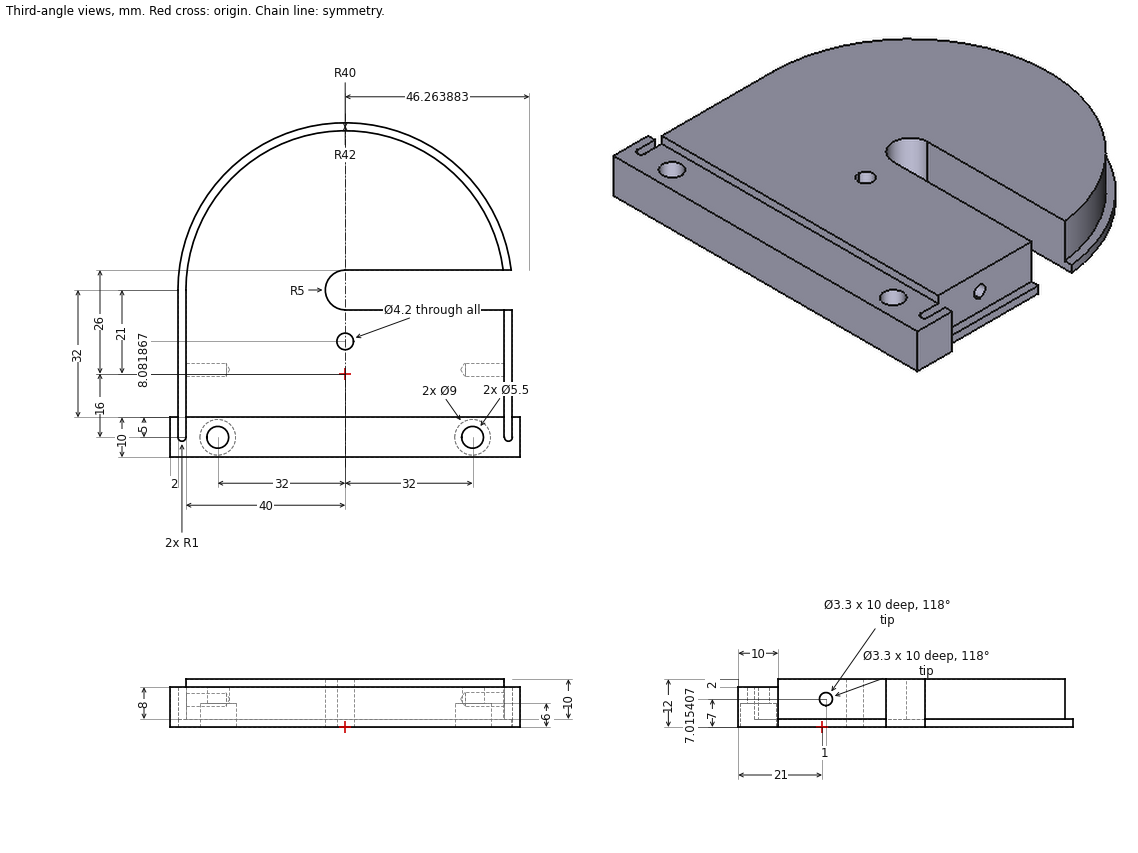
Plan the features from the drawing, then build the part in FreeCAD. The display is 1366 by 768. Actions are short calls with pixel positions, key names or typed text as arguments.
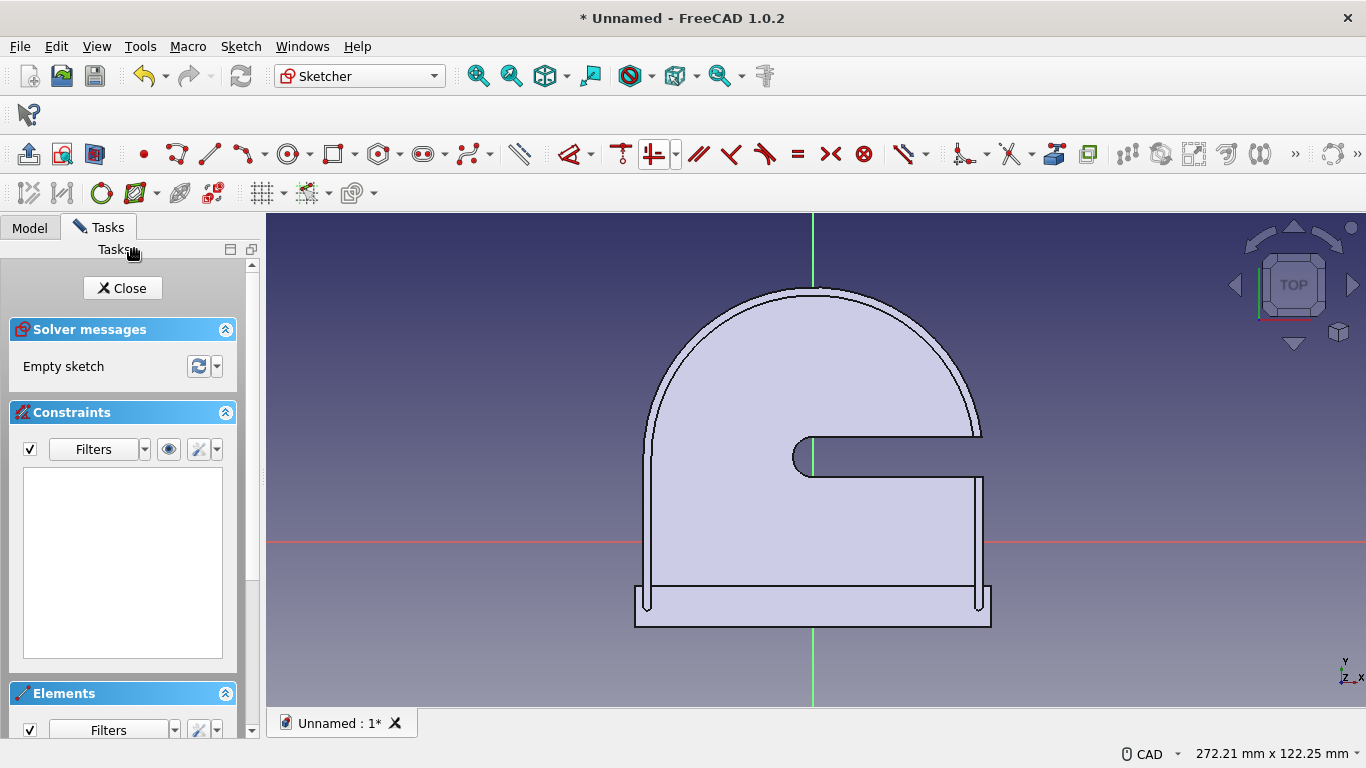
key(q)
key(s)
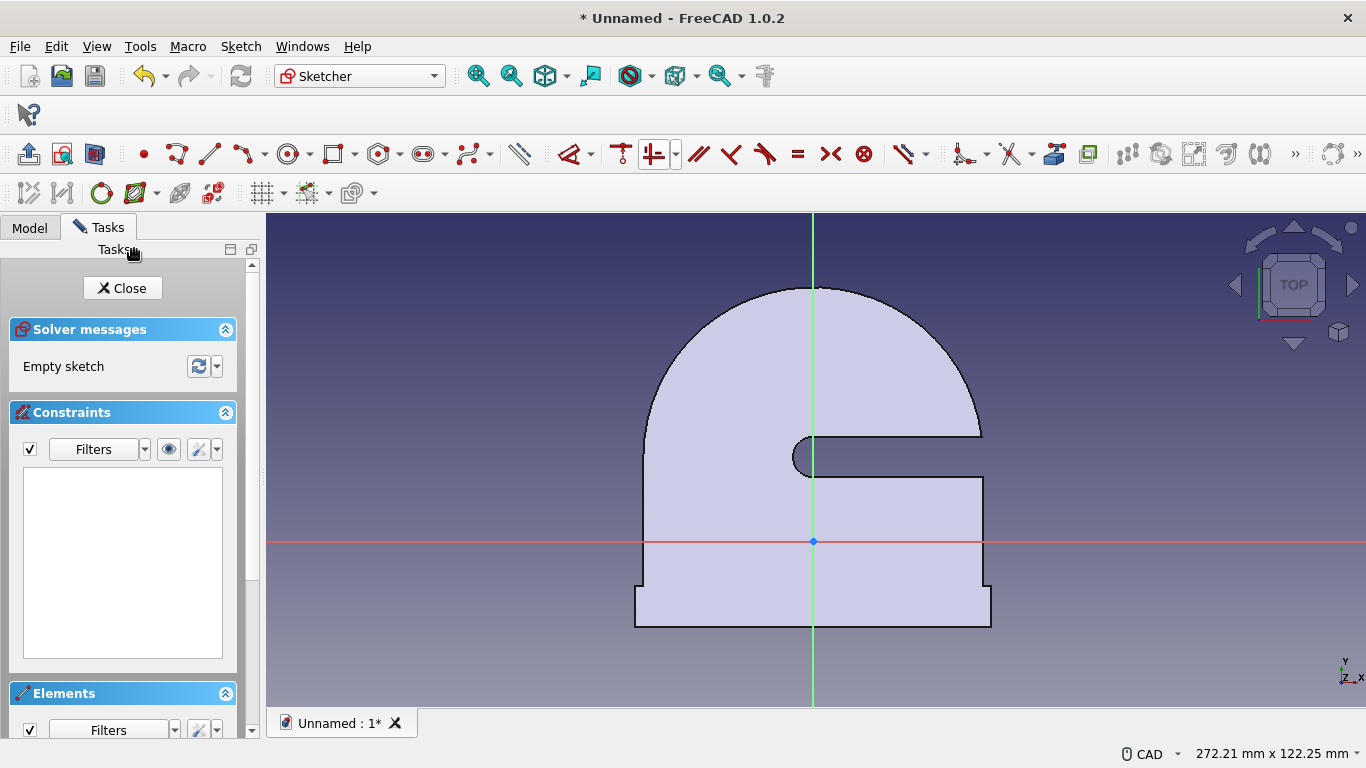
scroll(867, 677, up, 4)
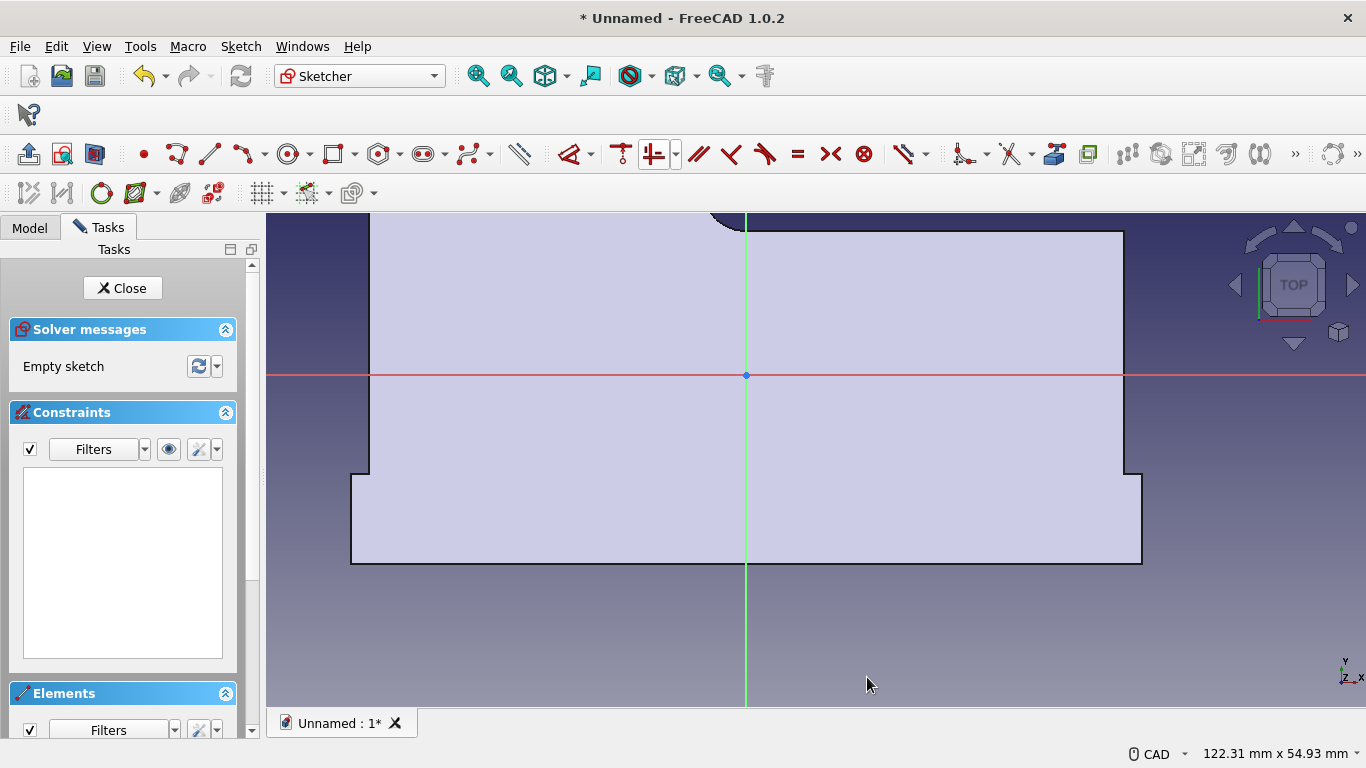
click(288, 154)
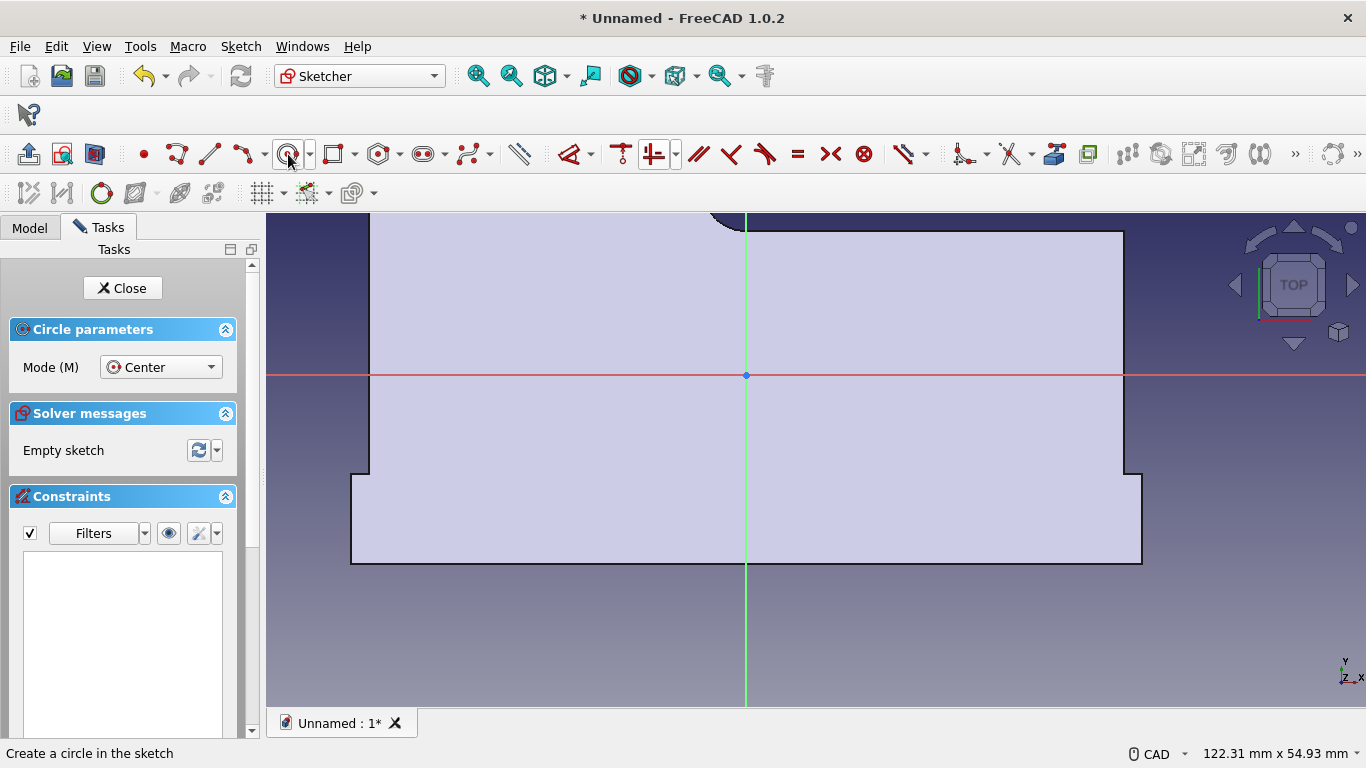
click(1034, 519)
click(1052, 502)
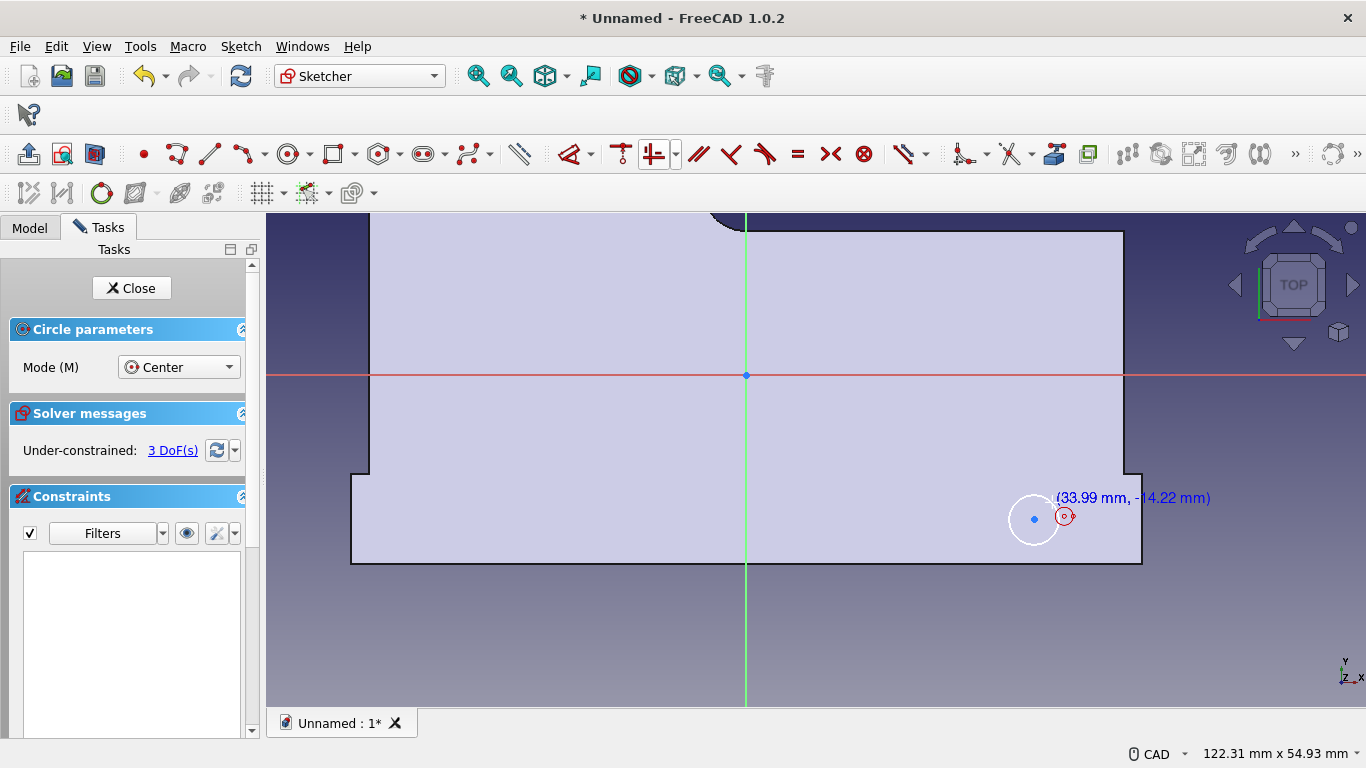
click(459, 519)
click(476, 502)
key(Escape)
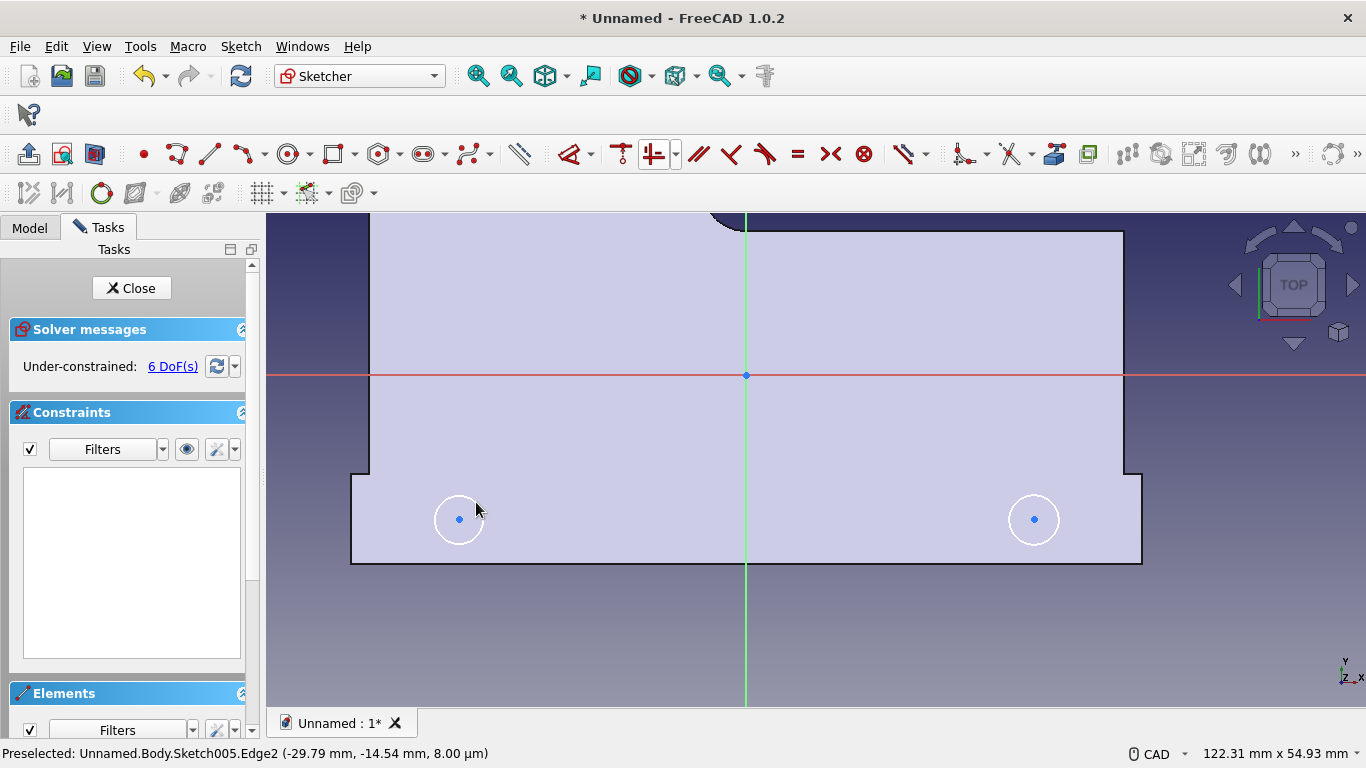
click(1051, 502)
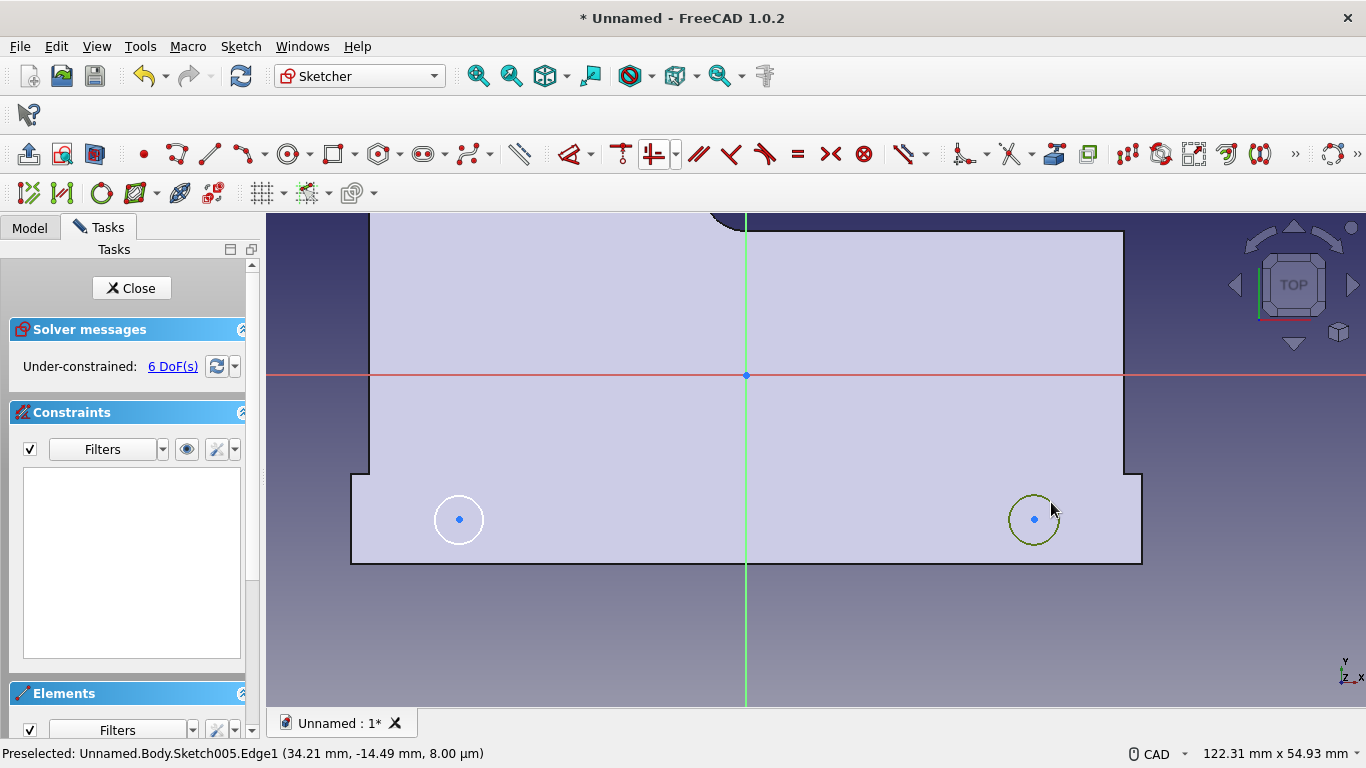
click(476, 503)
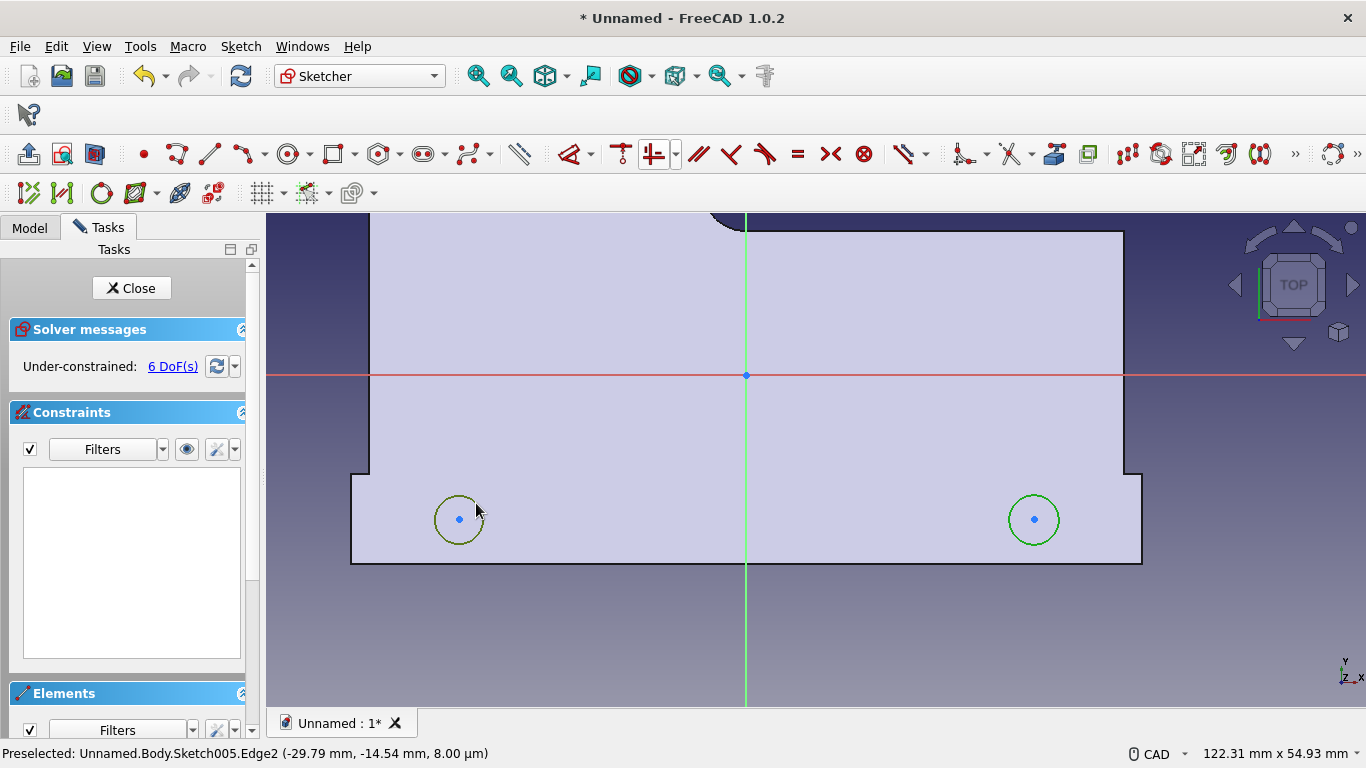
key(e)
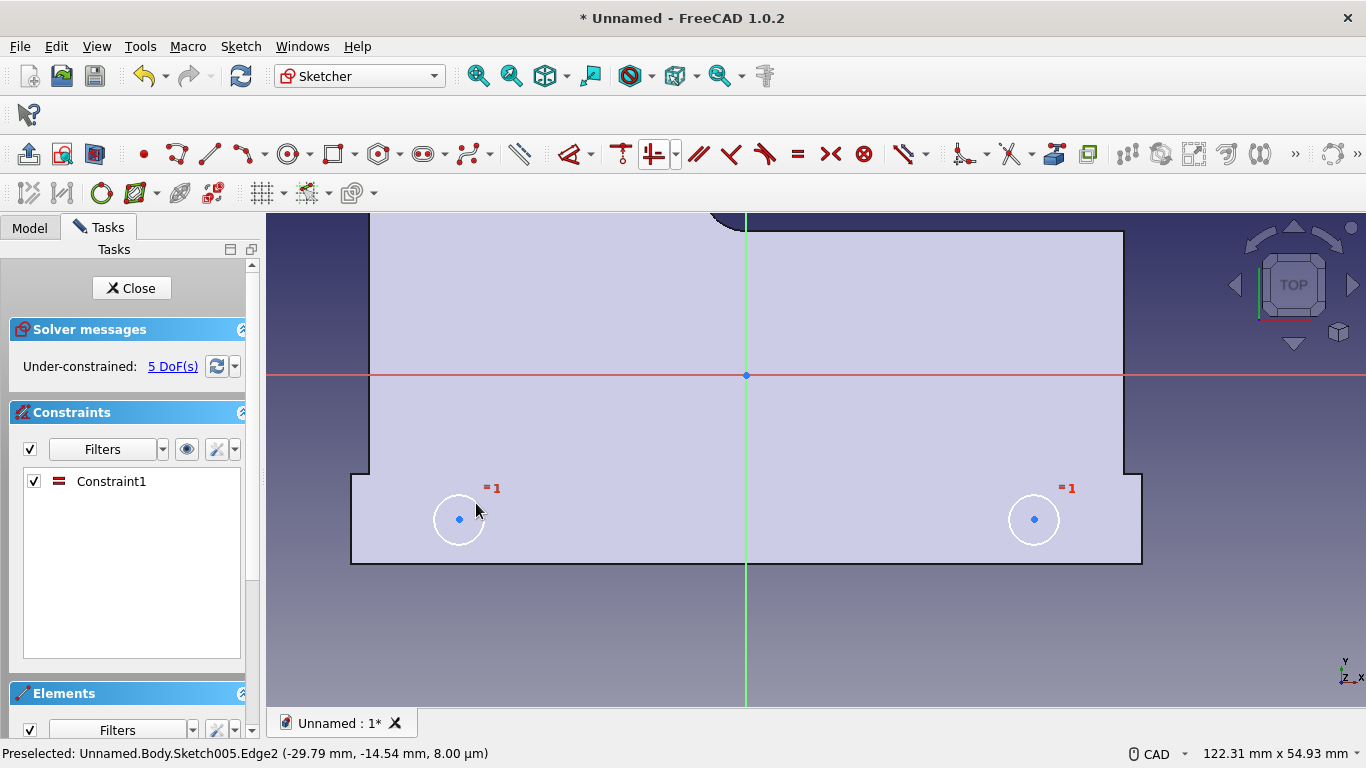
click(1034, 520)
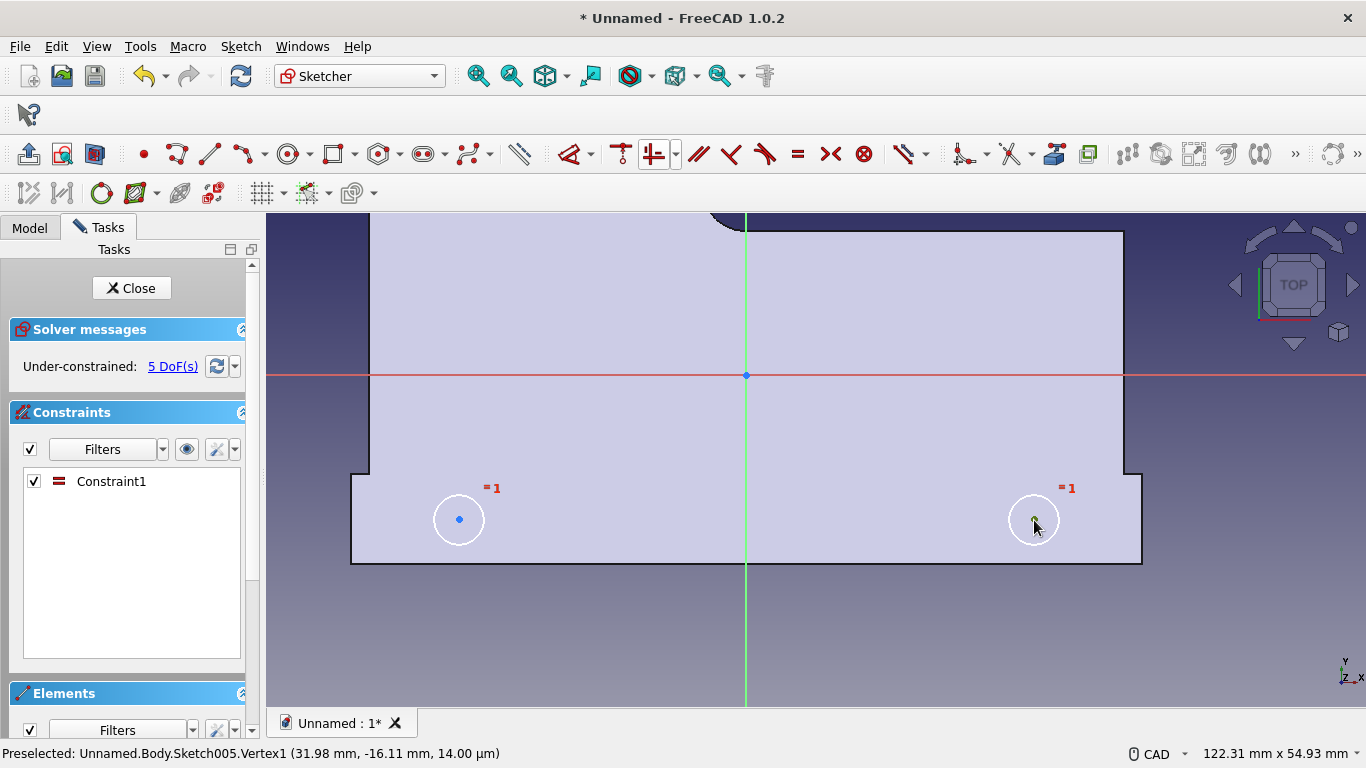
click(459, 520)